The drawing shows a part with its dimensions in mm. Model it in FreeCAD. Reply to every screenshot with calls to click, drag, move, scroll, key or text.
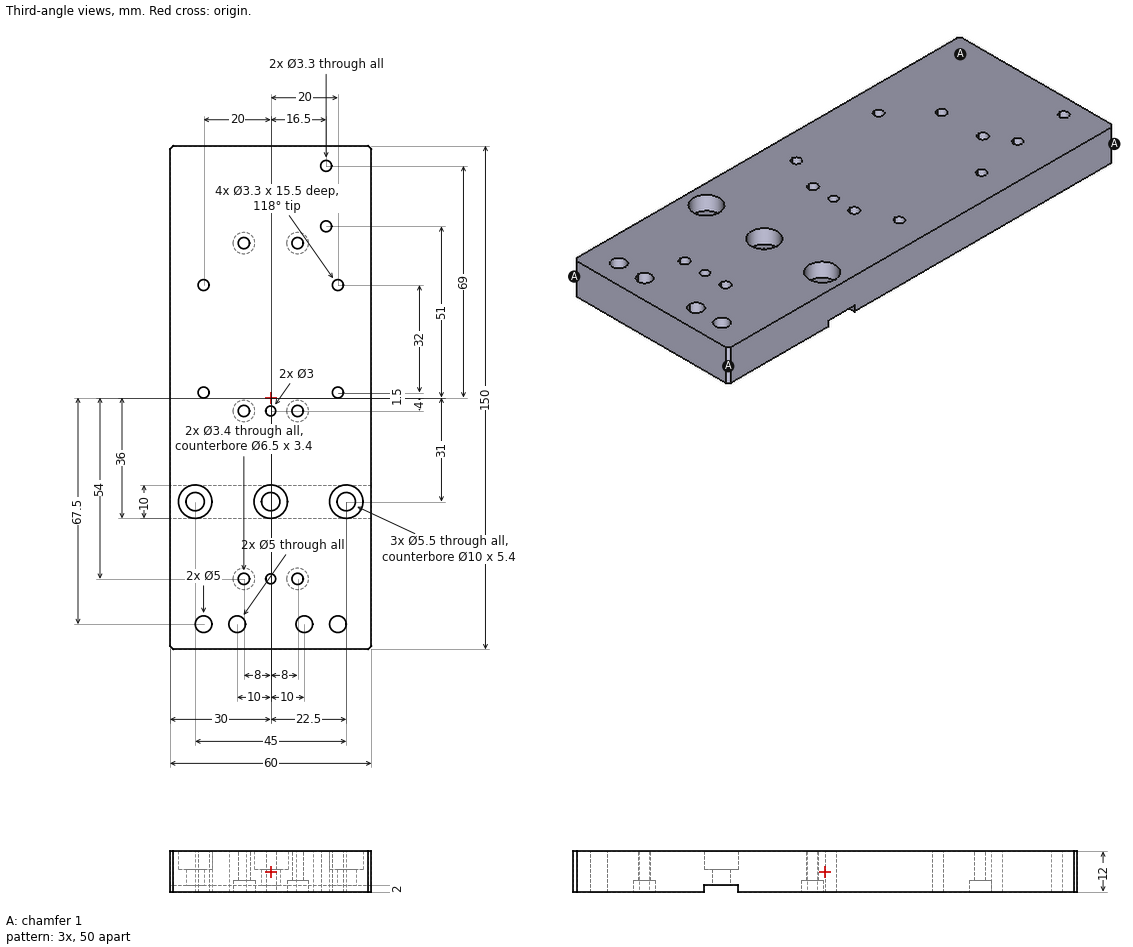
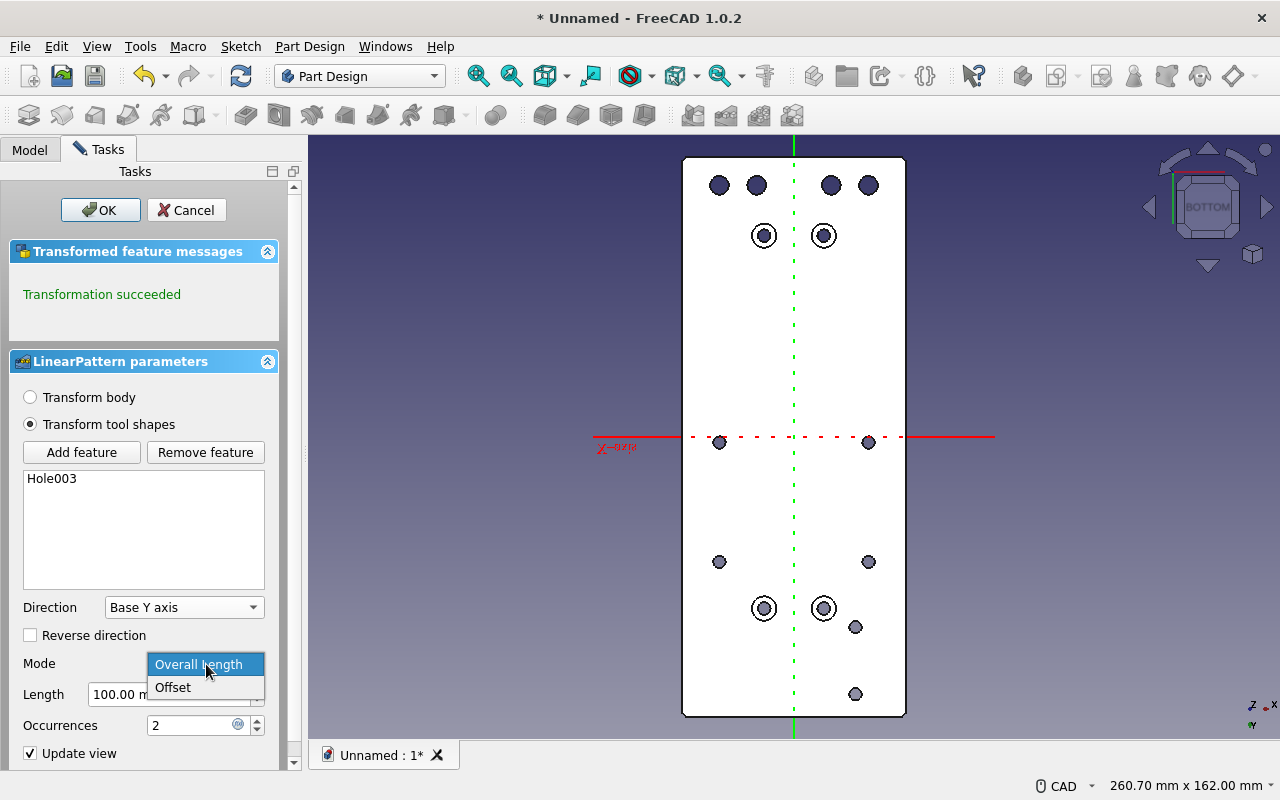
click(204, 688)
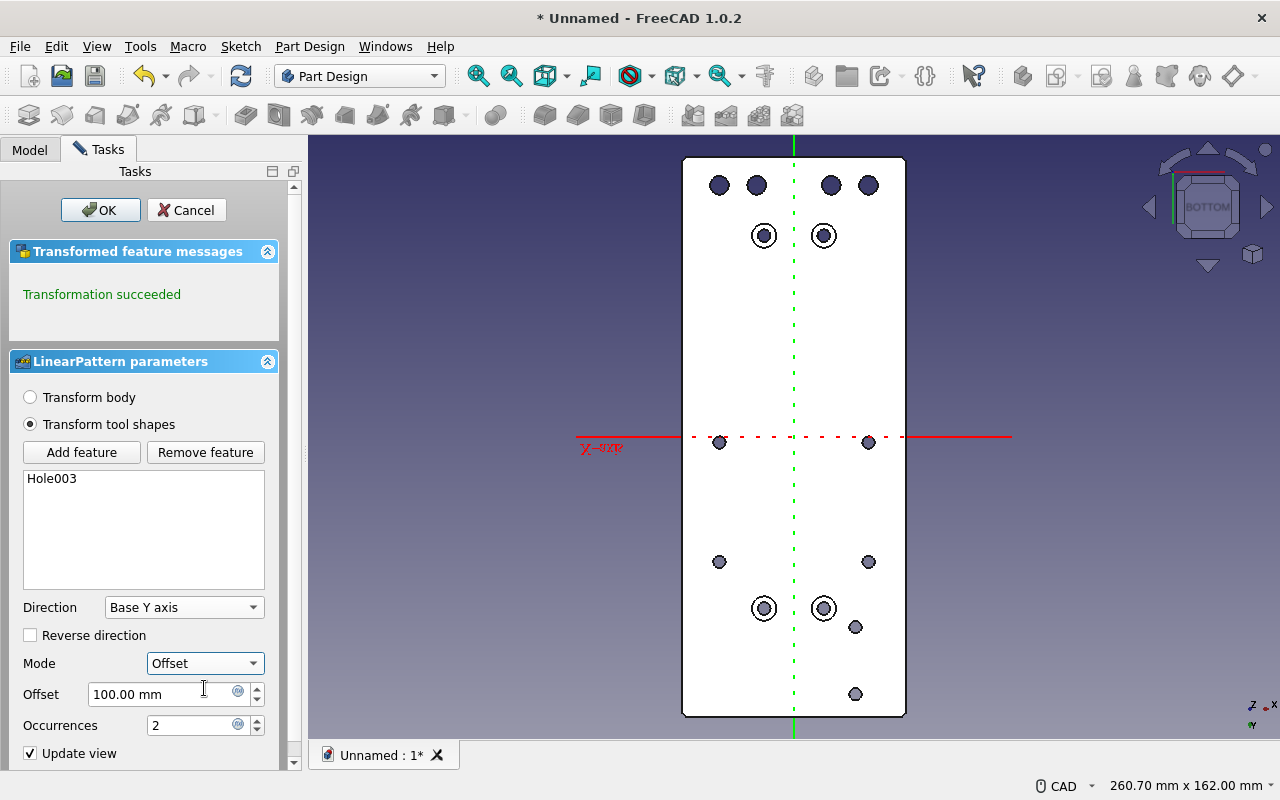
triple_click(170, 694)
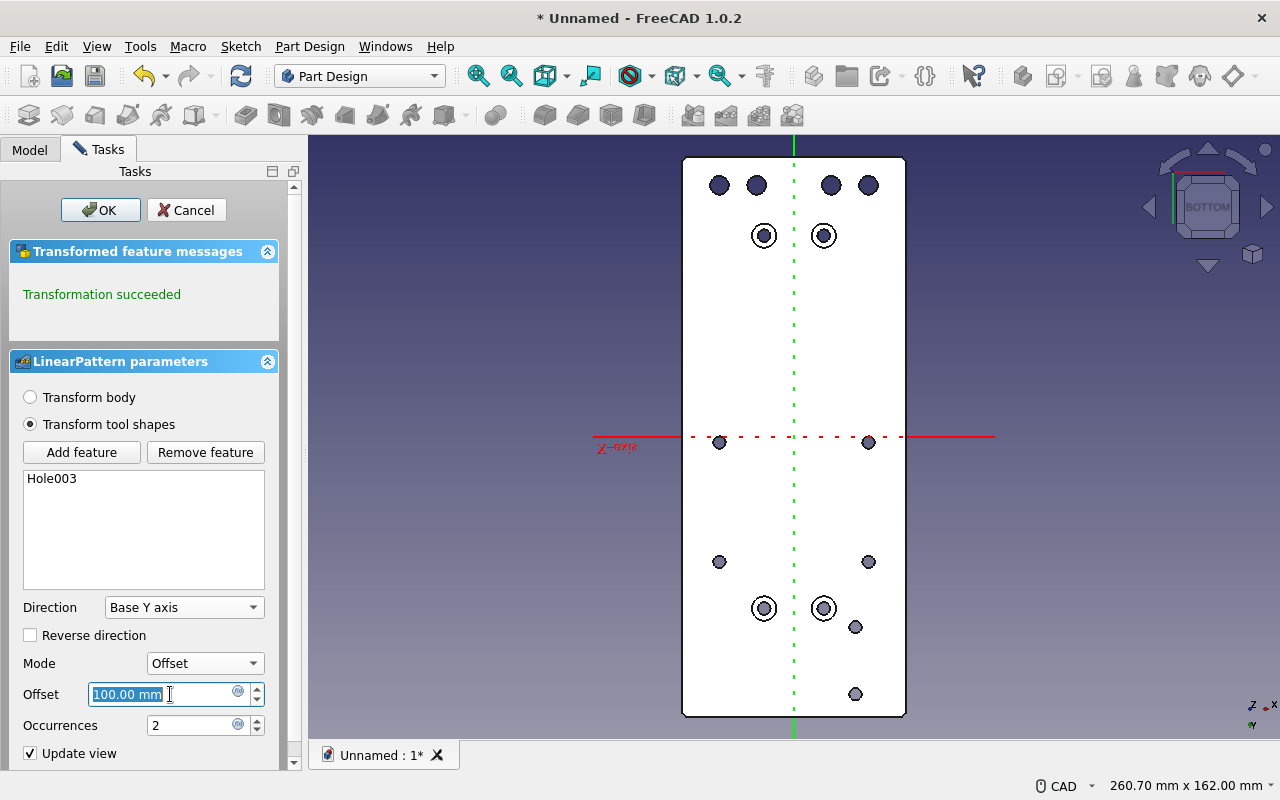
text(50)
key(Tab)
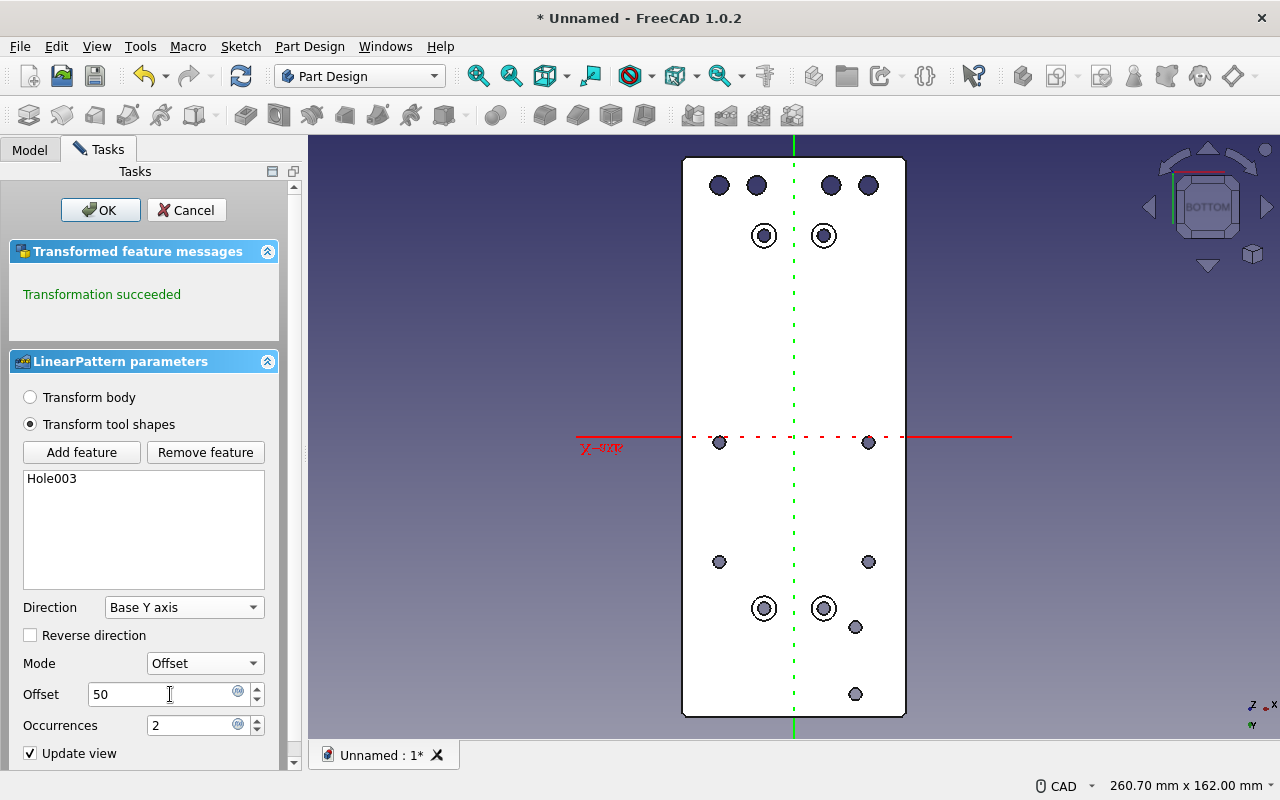
triple_click(199, 726)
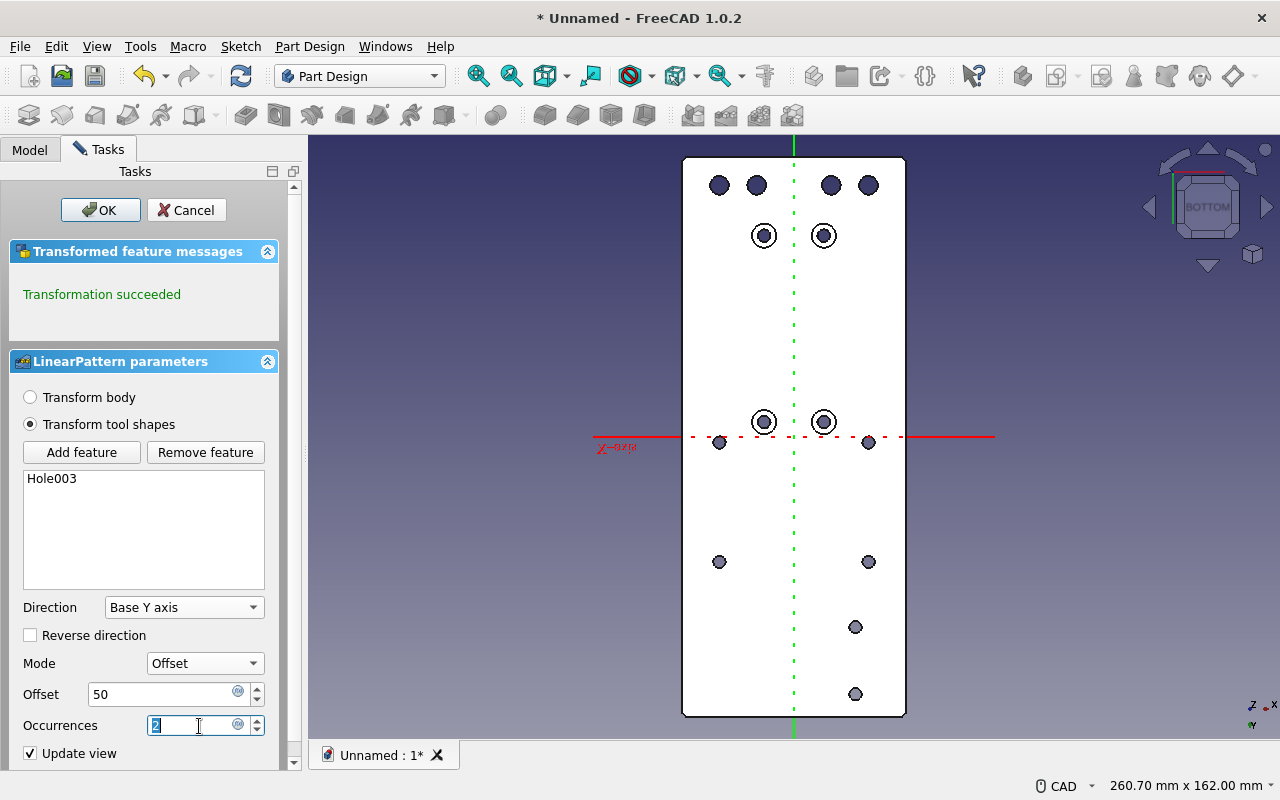
text(3)
key(Tab)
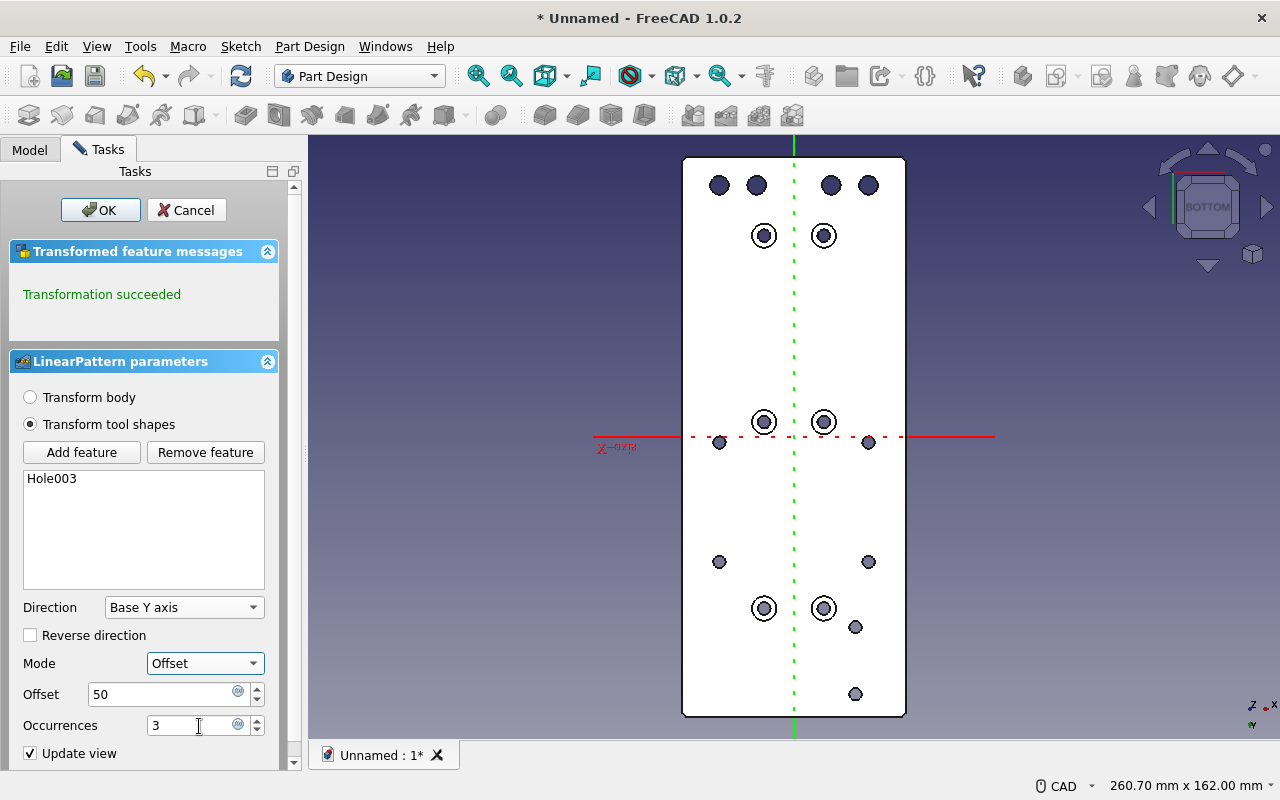
click(101, 210)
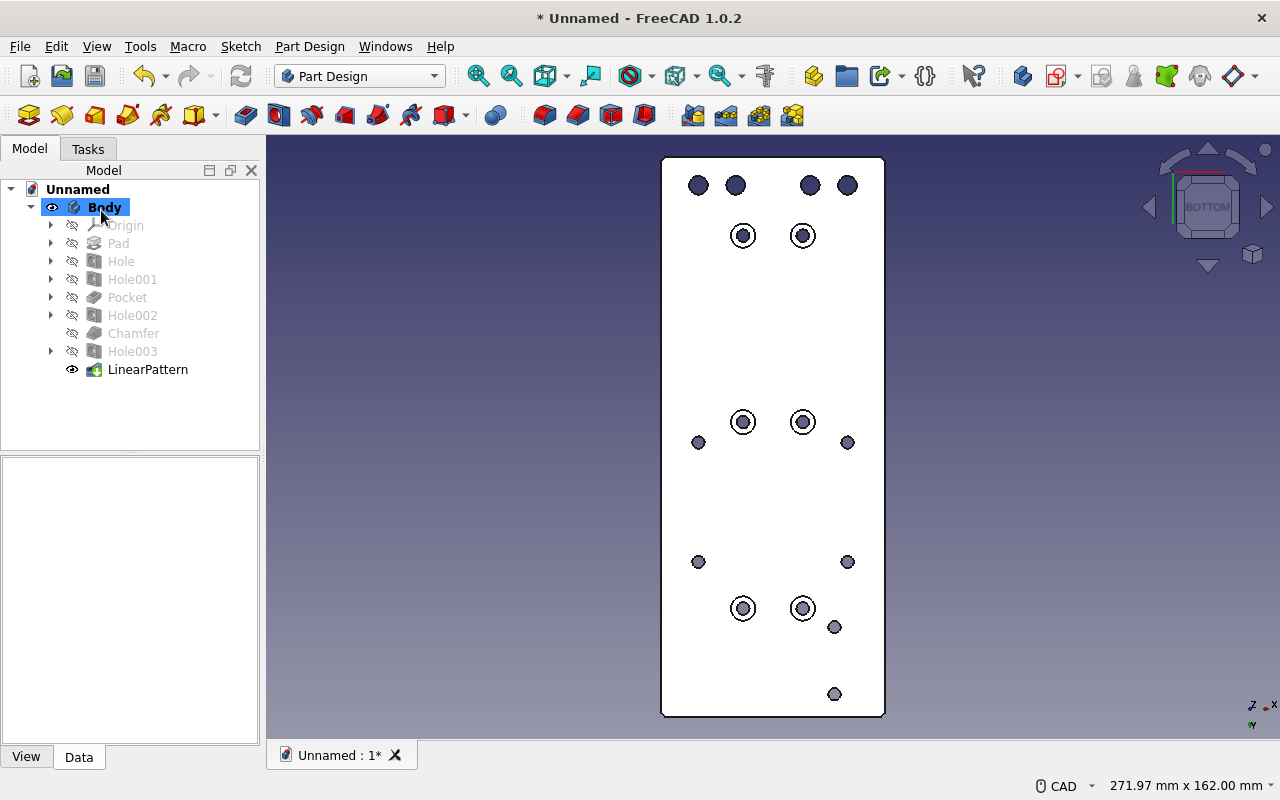
click(773, 516)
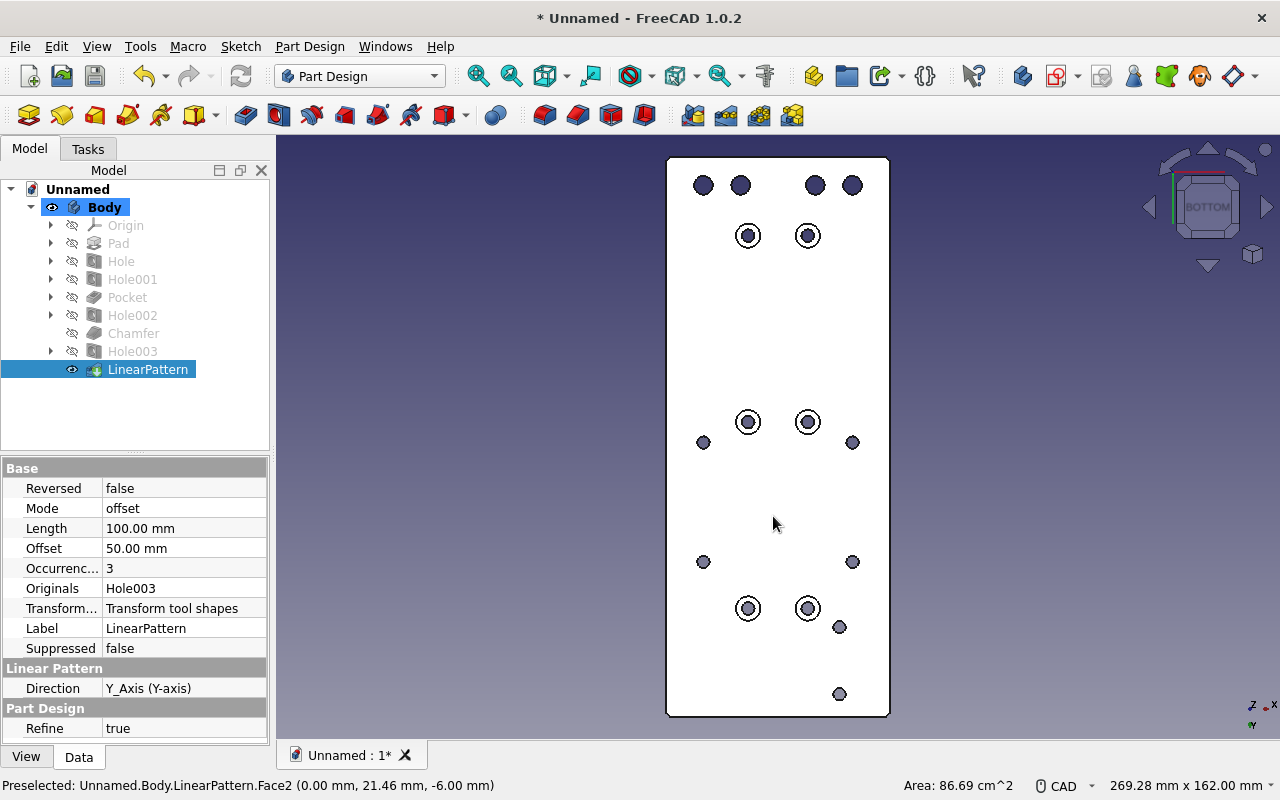
click(1056, 76)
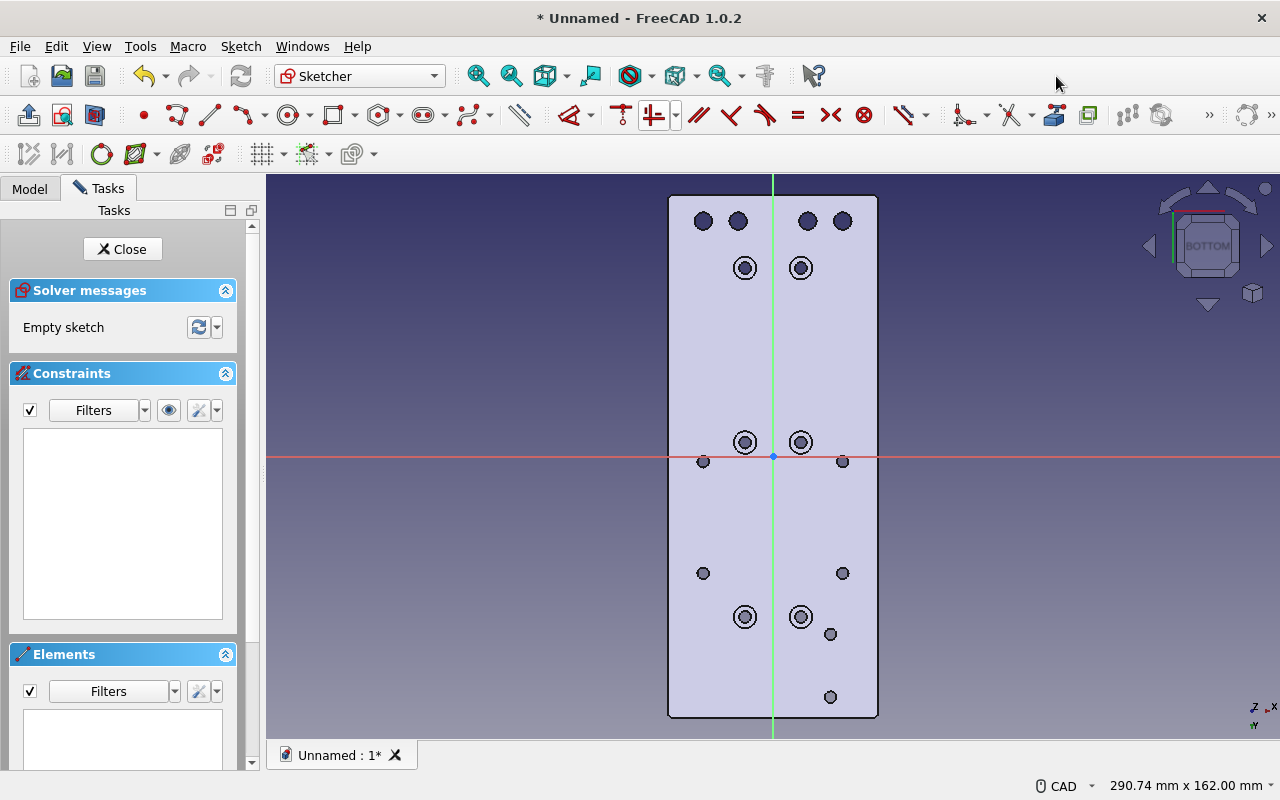
scroll(856, 242, up, 3)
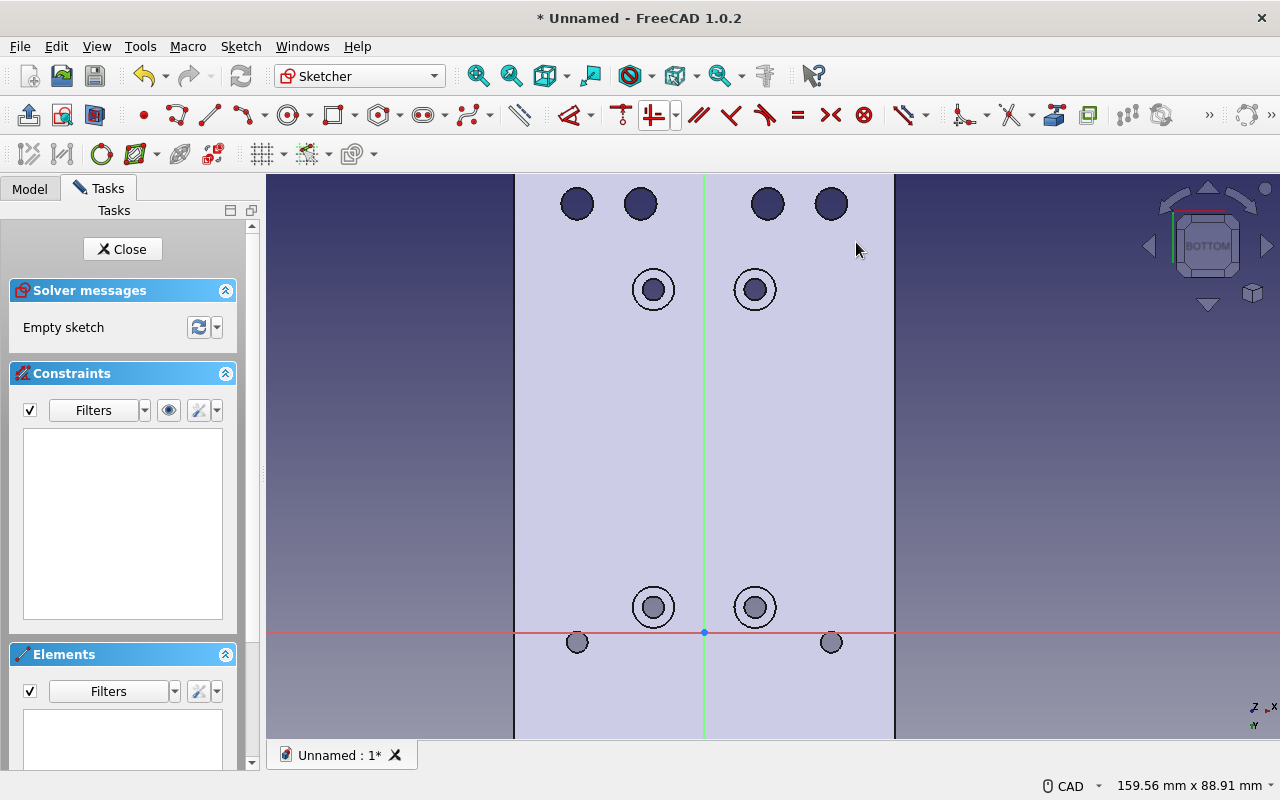
click(288, 116)